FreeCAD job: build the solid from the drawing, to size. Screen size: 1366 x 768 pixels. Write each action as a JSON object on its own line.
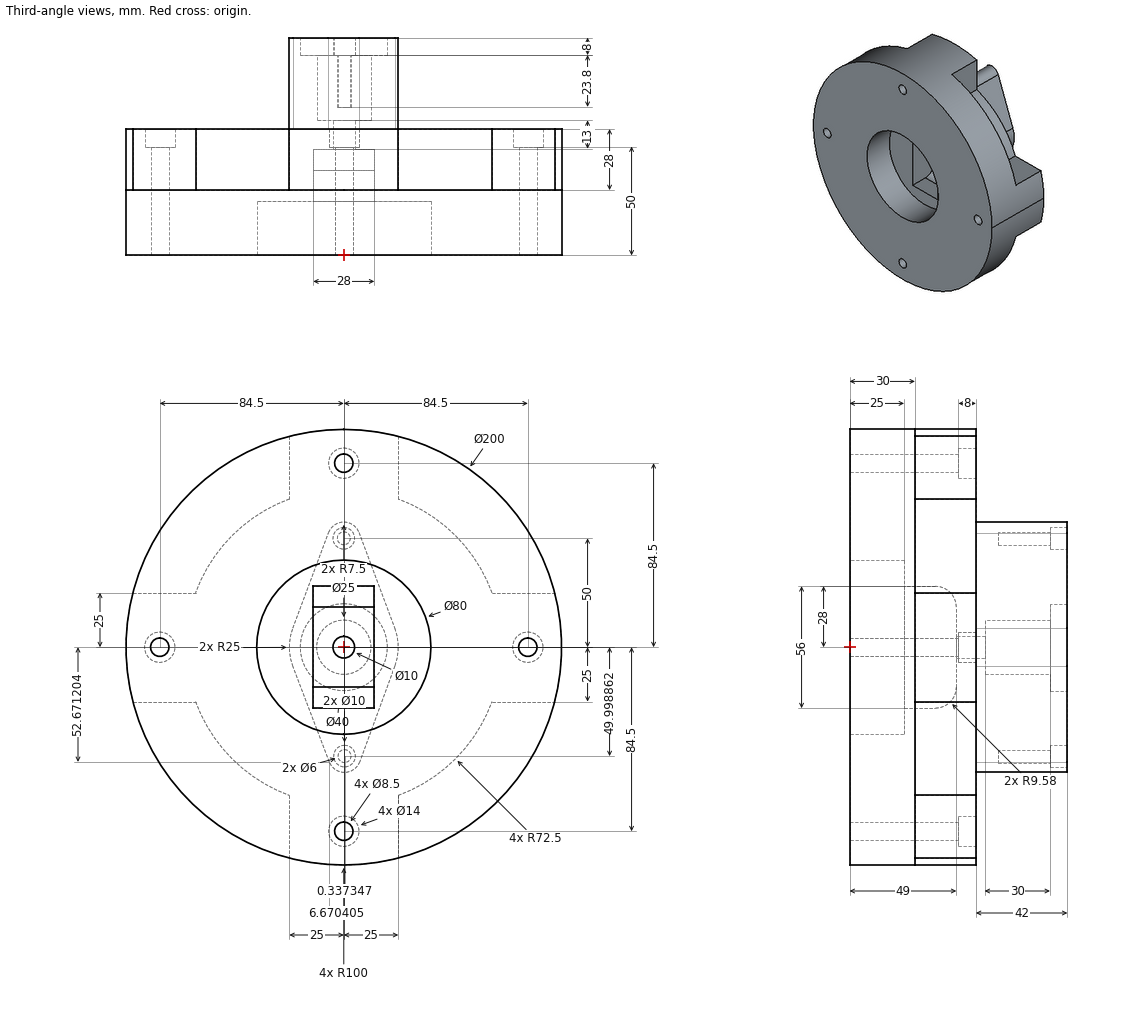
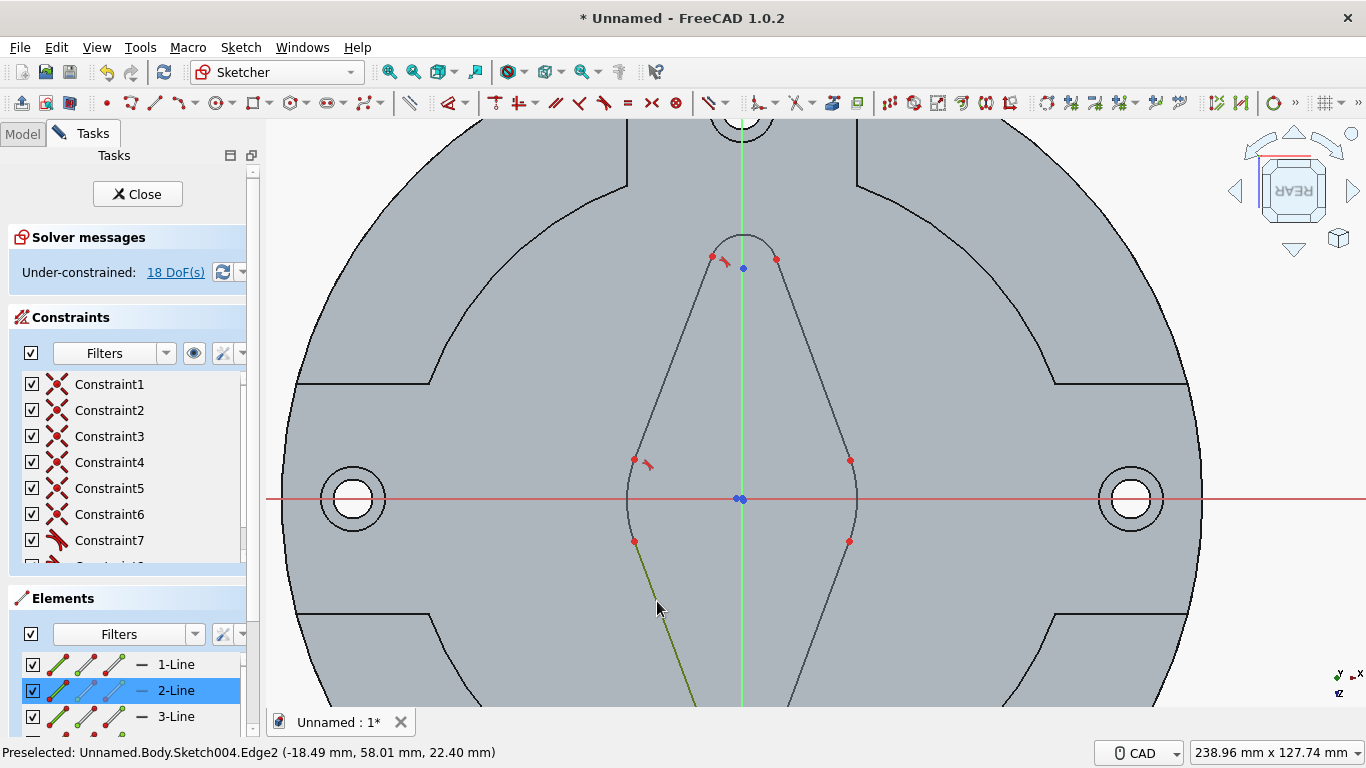
{"action": "left_click", "coordinate": [628, 483]}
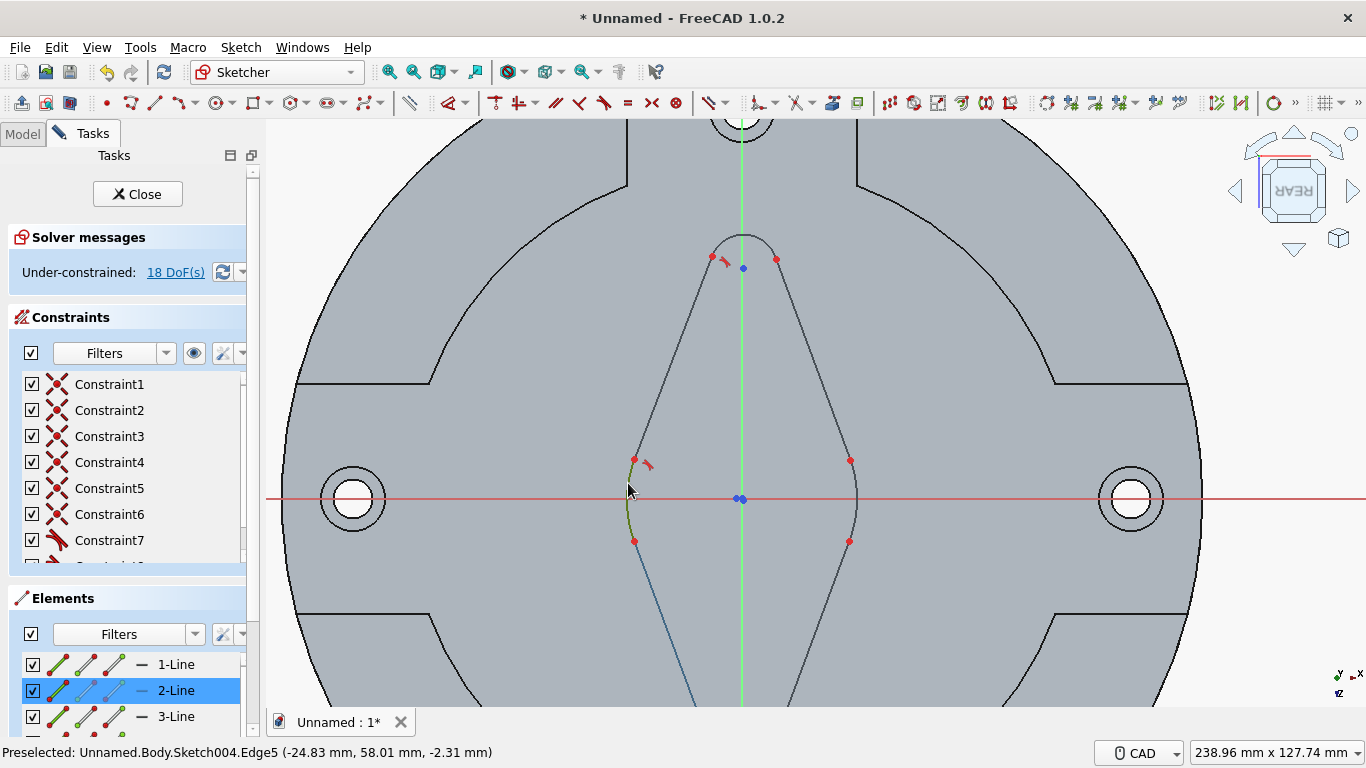
{"action": "key", "text": "t"}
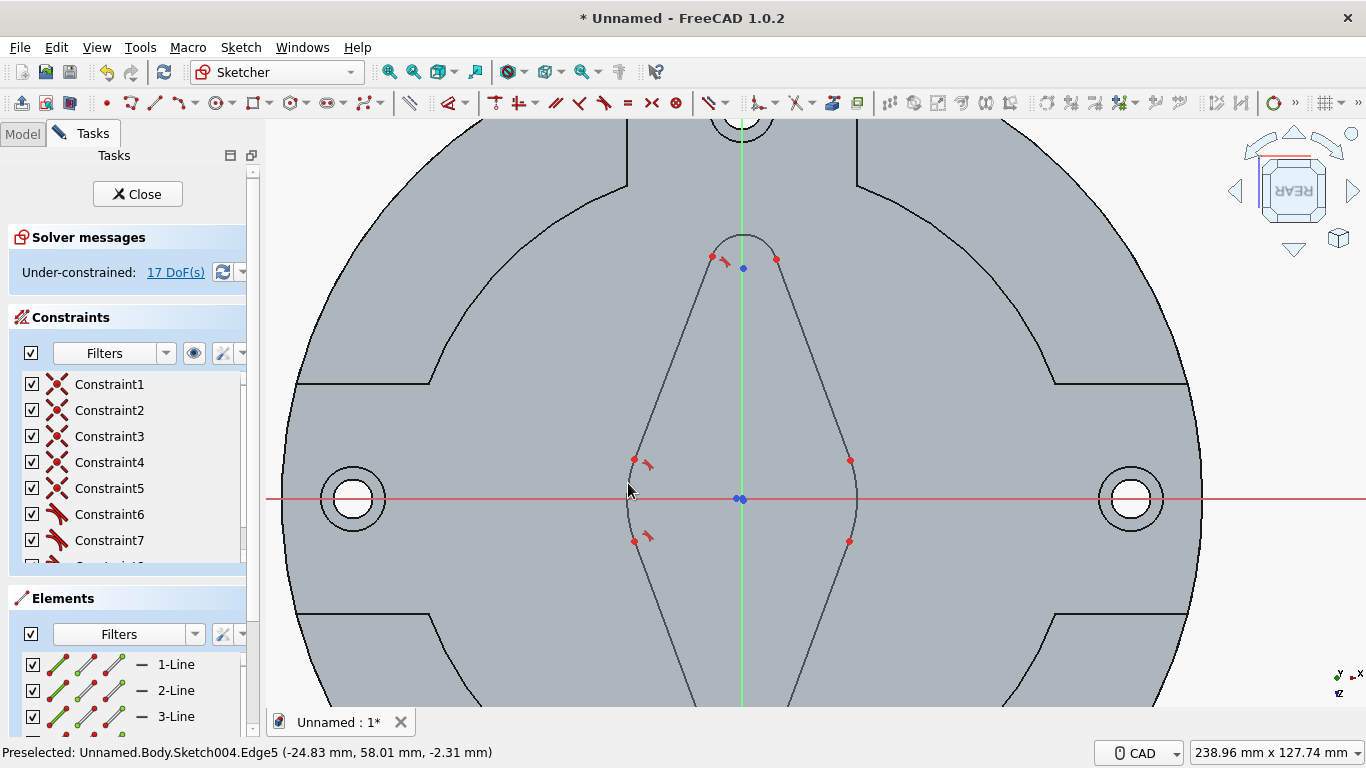
{"action": "left_click", "coordinate": [657, 601]}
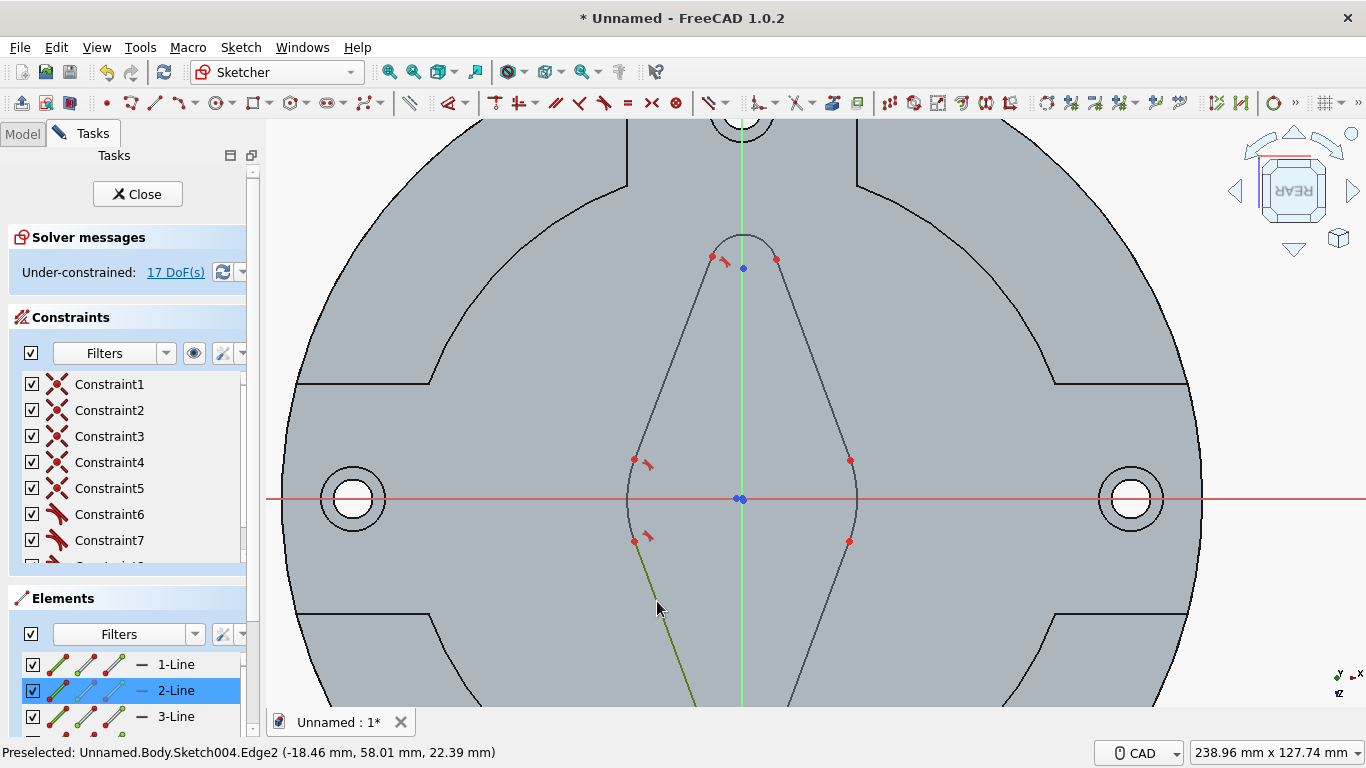
{"action": "scroll", "coordinate": [759, 238], "scroll_direction": "down", "scroll_amount": 2}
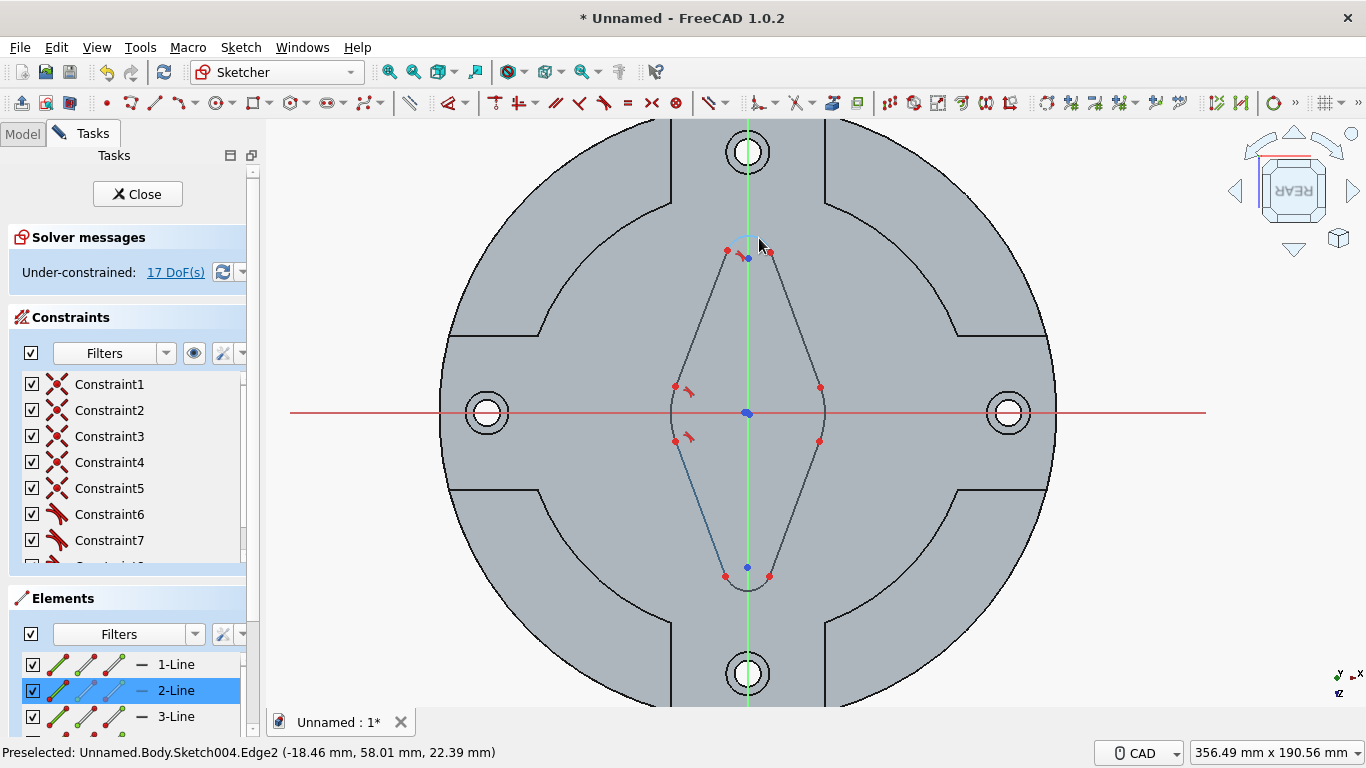
{"action": "scroll", "coordinate": [737, 588], "scroll_direction": "up", "scroll_amount": 2}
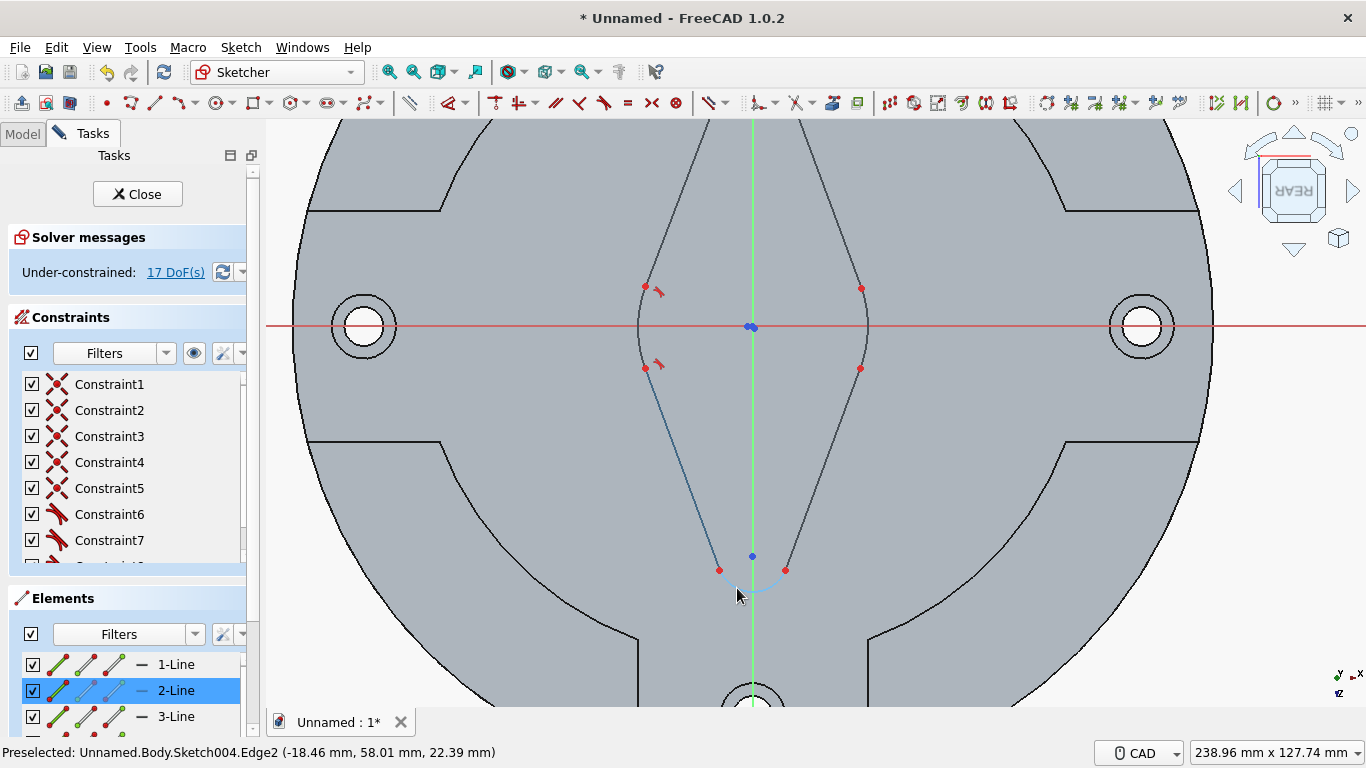
{"action": "left_click", "coordinate": [737, 588]}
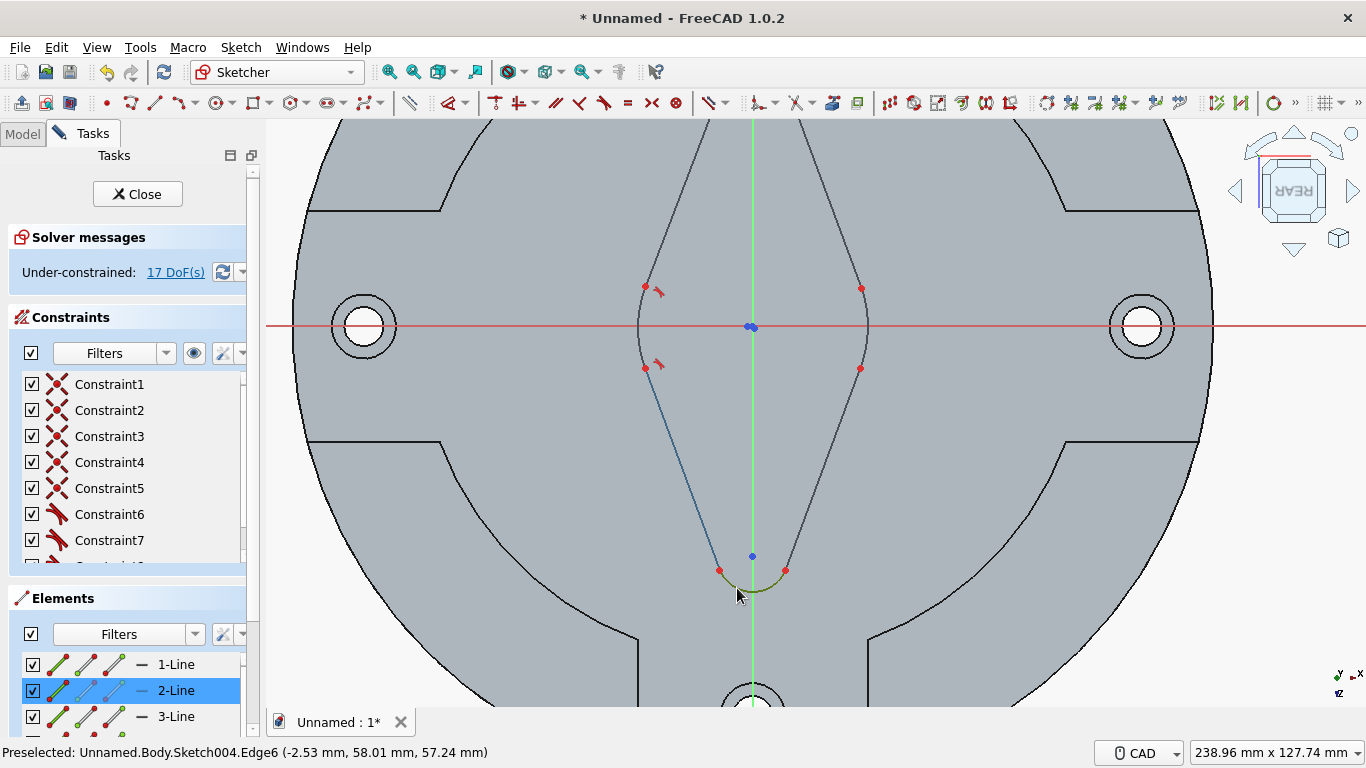
{"action": "key", "text": "t"}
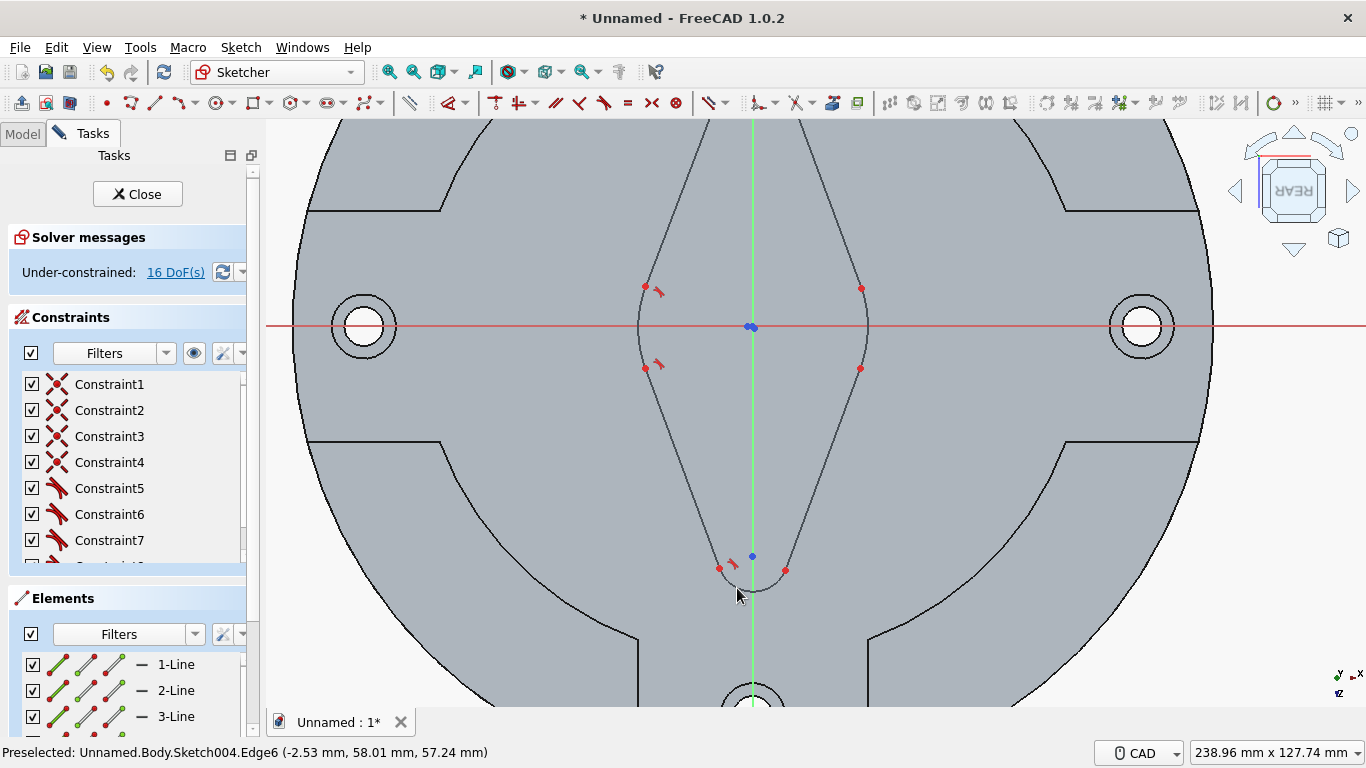
{"action": "left_click", "coordinate": [808, 510]}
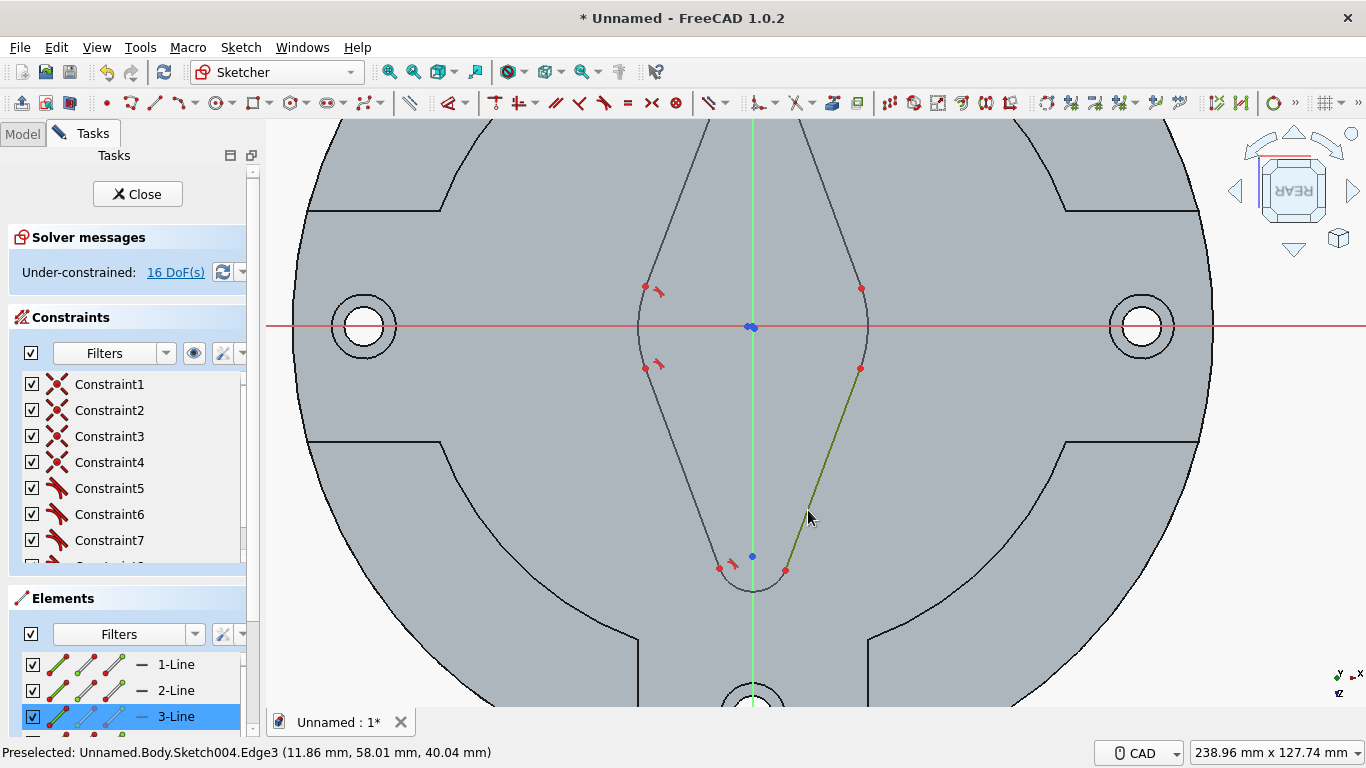
{"action": "left_click", "coordinate": [736, 587]}